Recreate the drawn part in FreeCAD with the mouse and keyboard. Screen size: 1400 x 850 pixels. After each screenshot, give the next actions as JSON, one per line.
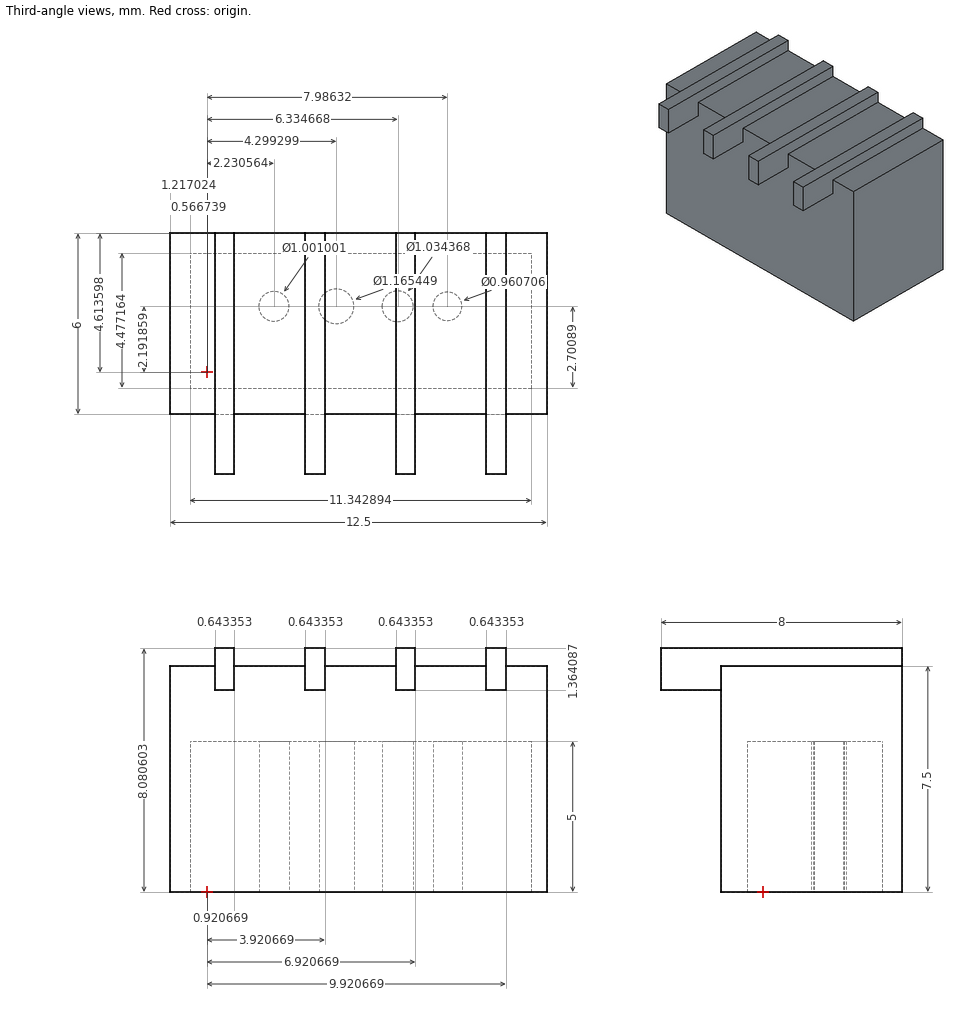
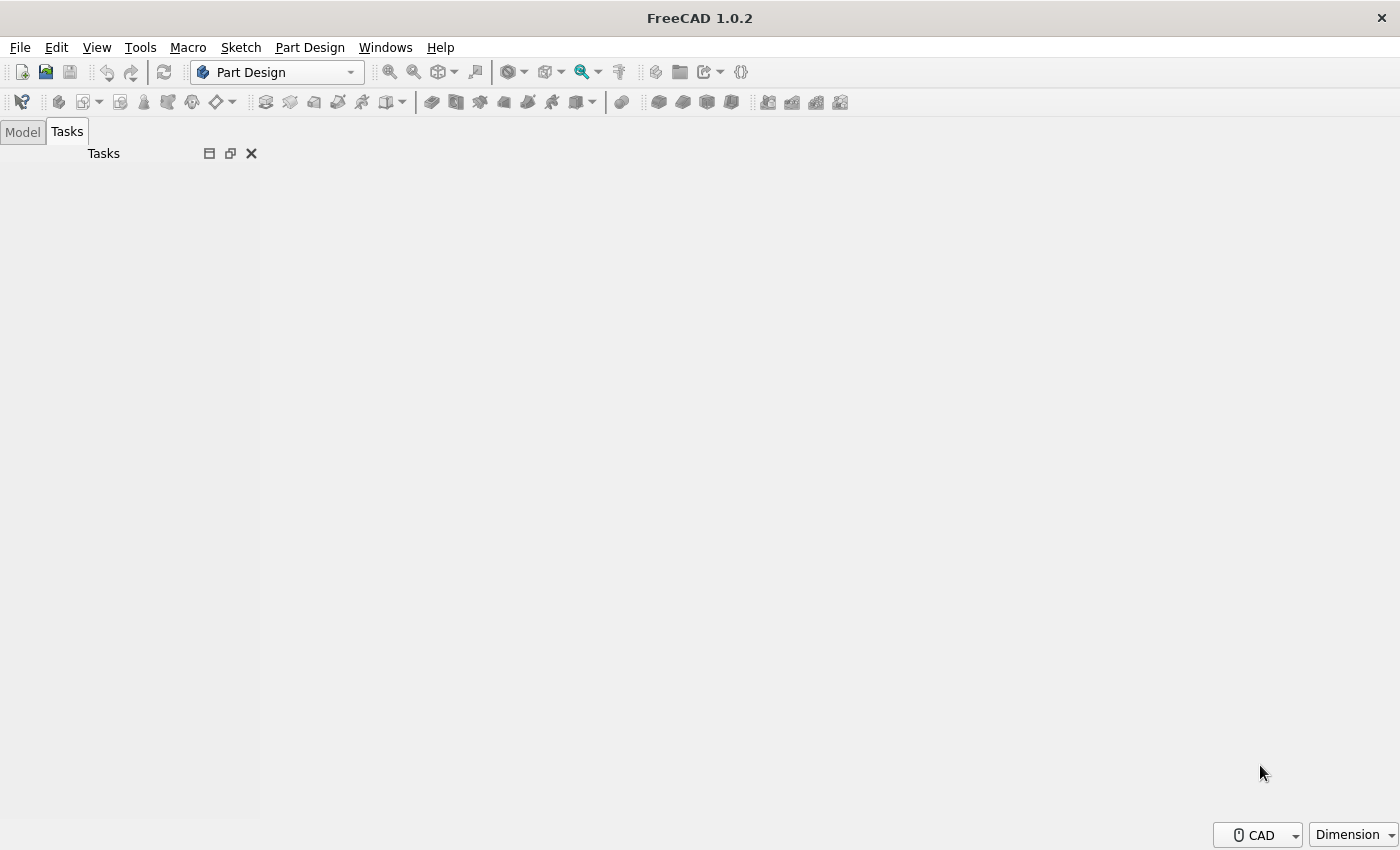
{"action": "key", "text": "ctrl+n"}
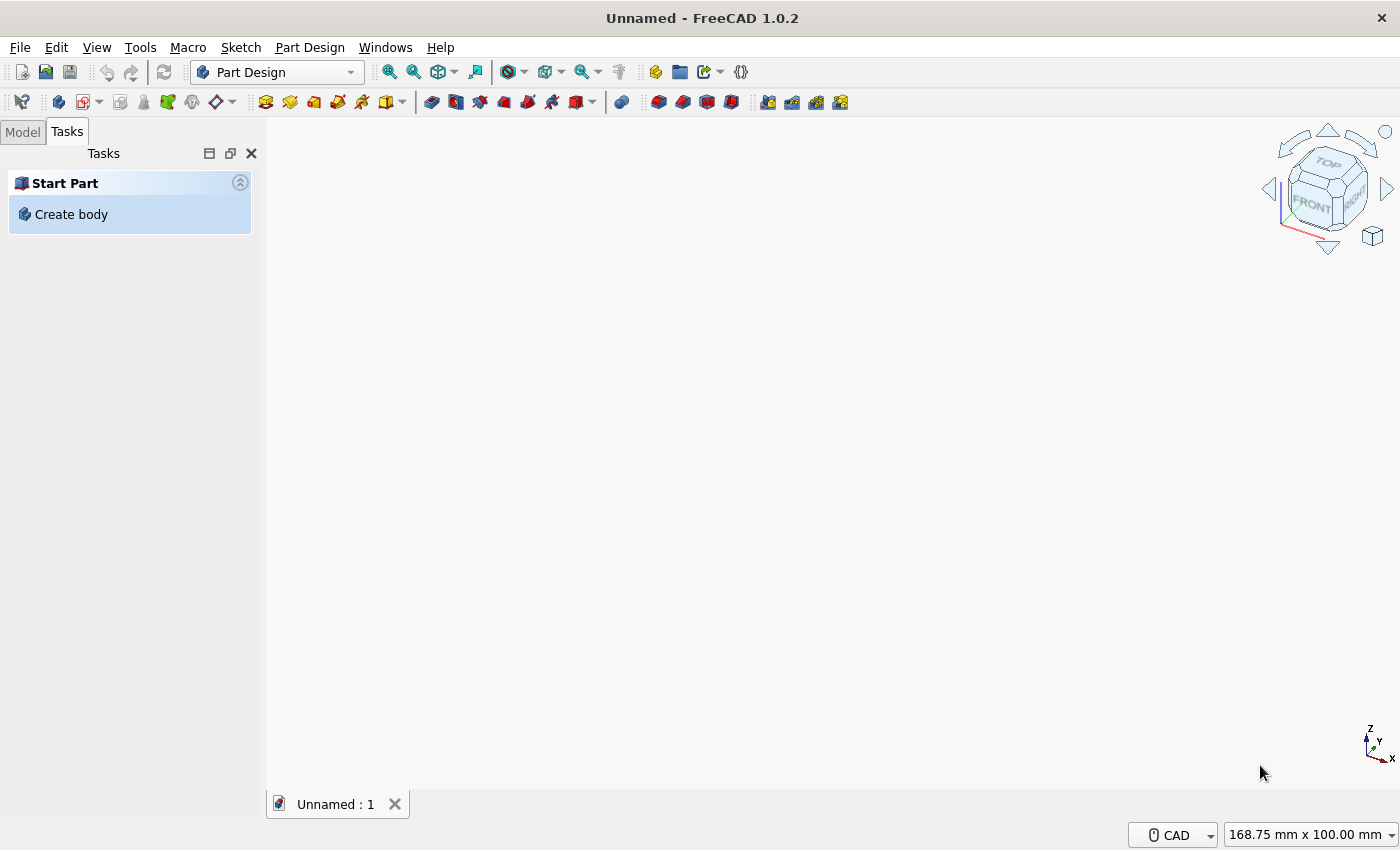
{"action": "left_click", "coordinate": [84, 102]}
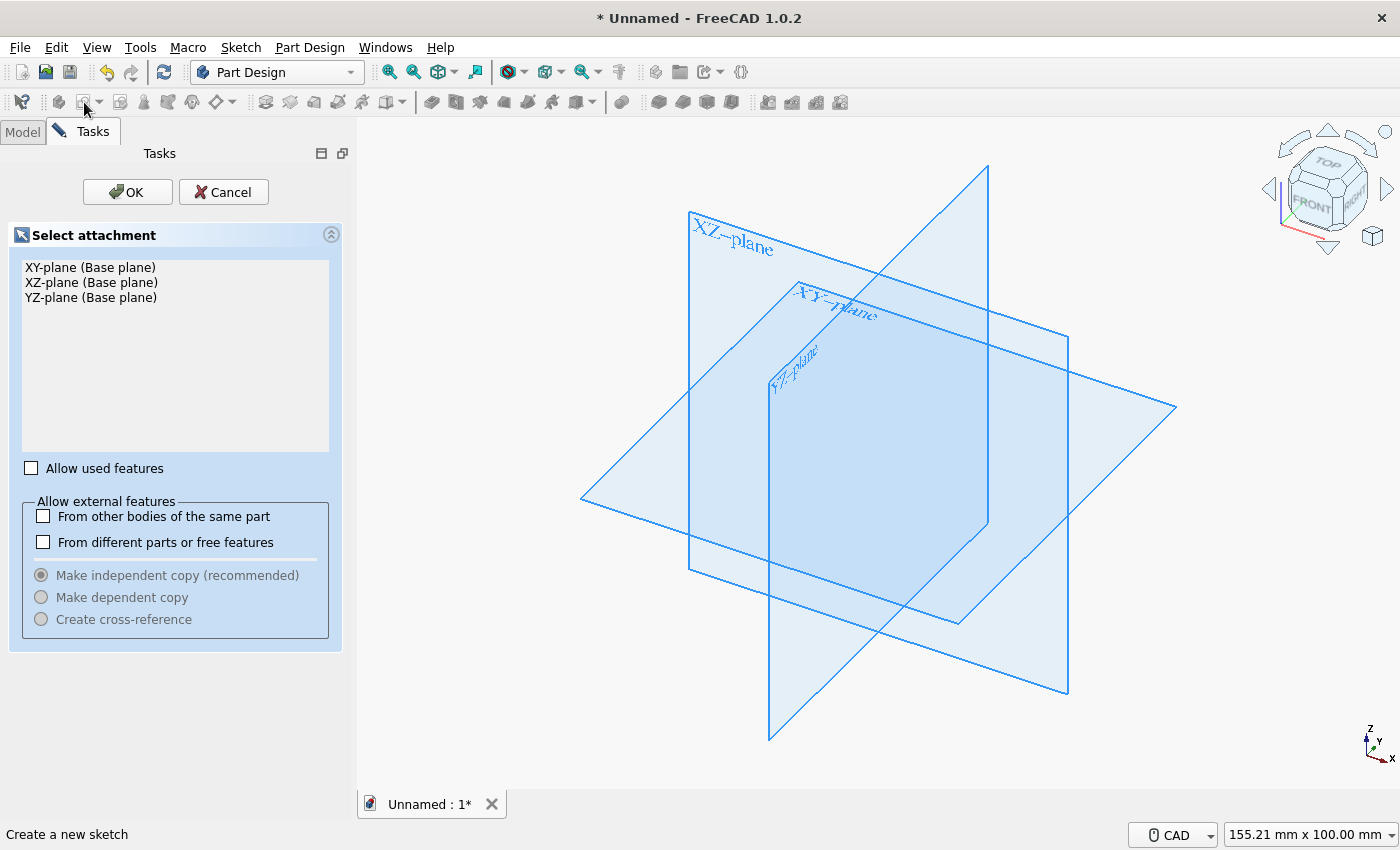
{"action": "left_click", "coordinate": [82, 268]}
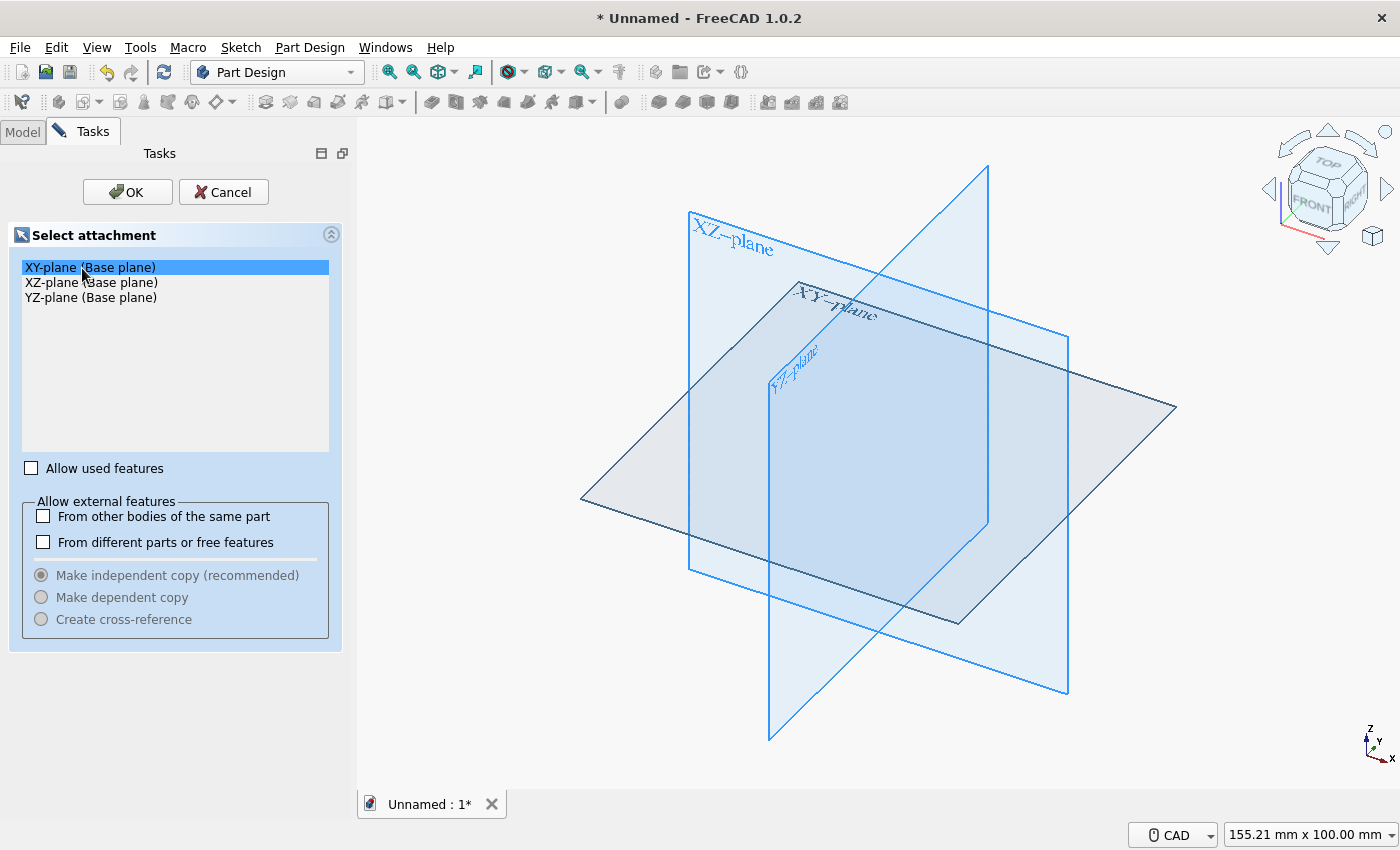
{"action": "left_click", "coordinate": [128, 192]}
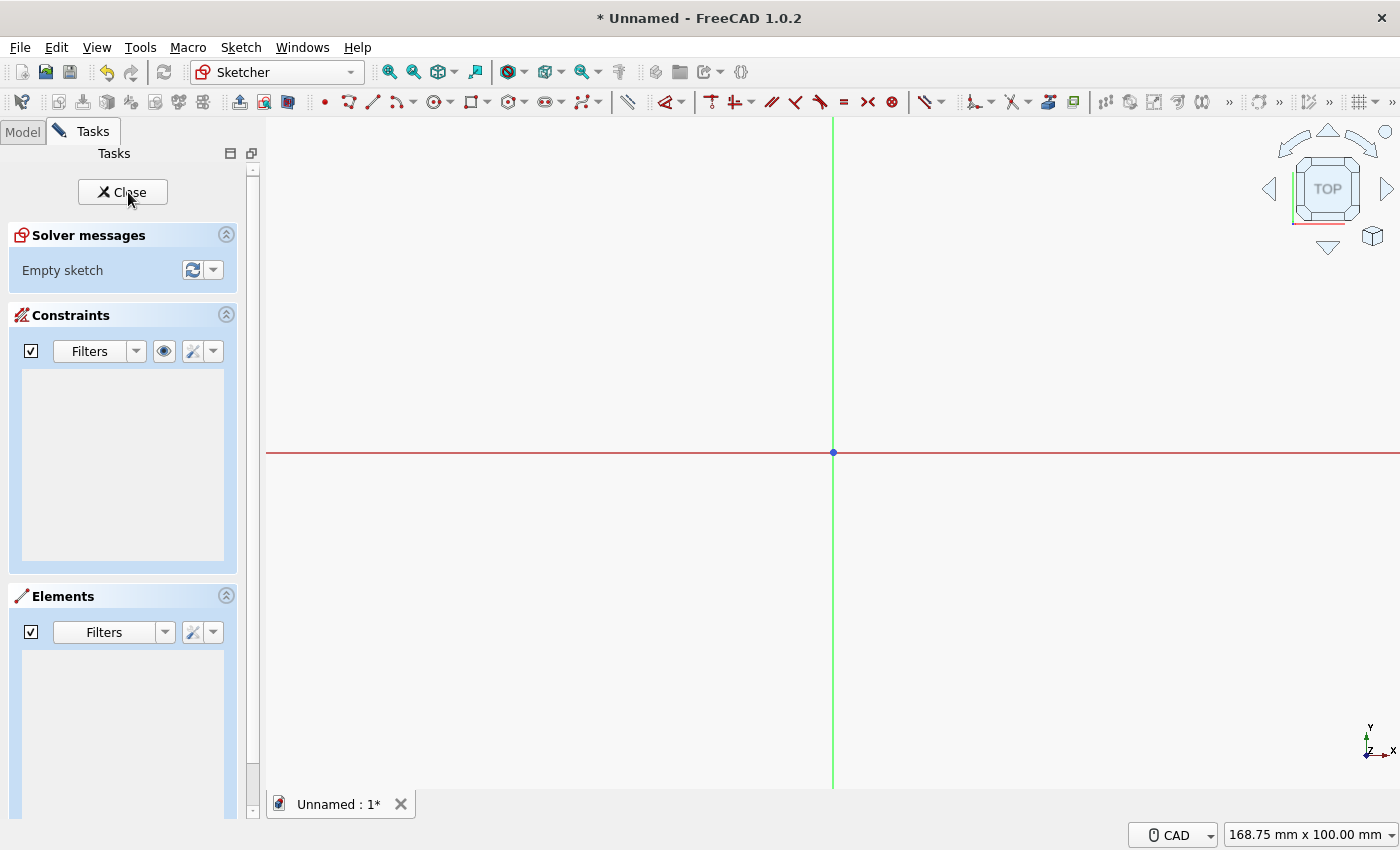
{"action": "scroll", "coordinate": [883, 440], "scroll_direction": "up", "scroll_amount": 10}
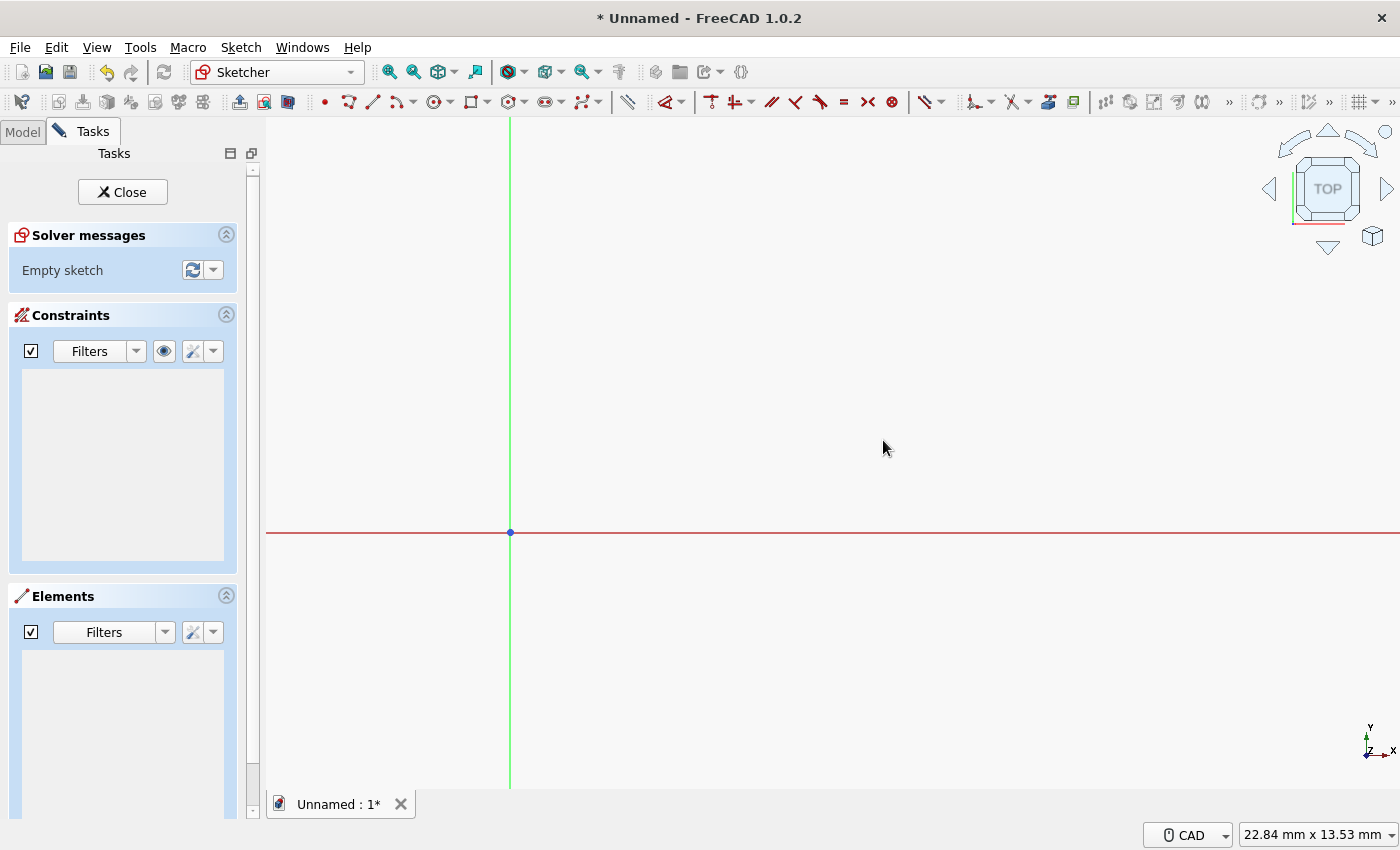
{"action": "key", "text": "g r"}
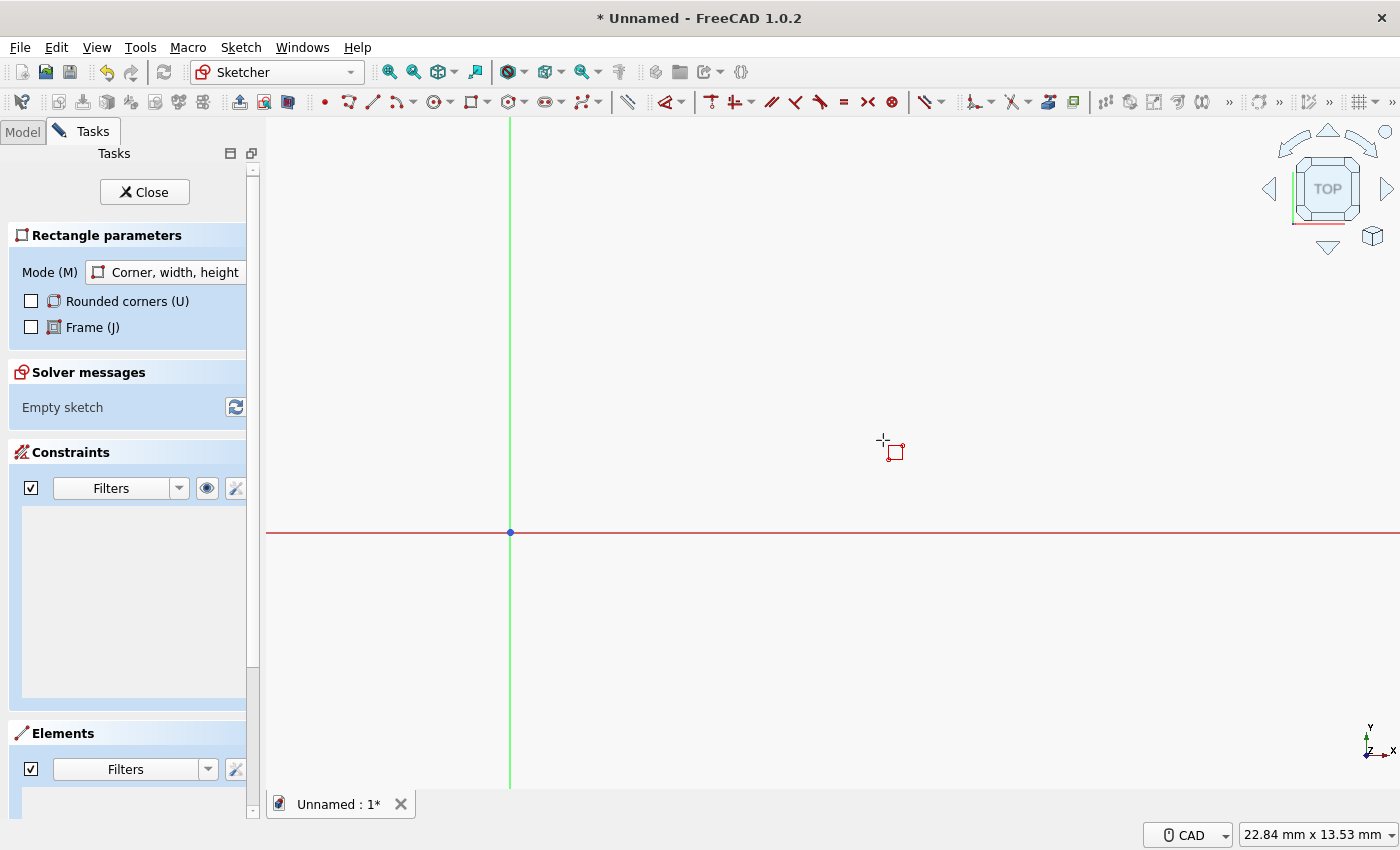
{"action": "left_click", "coordinate": [450, 304]}
{"action": "left_click", "coordinate": [1070, 602]}
{"action": "key", "text": "Escape"}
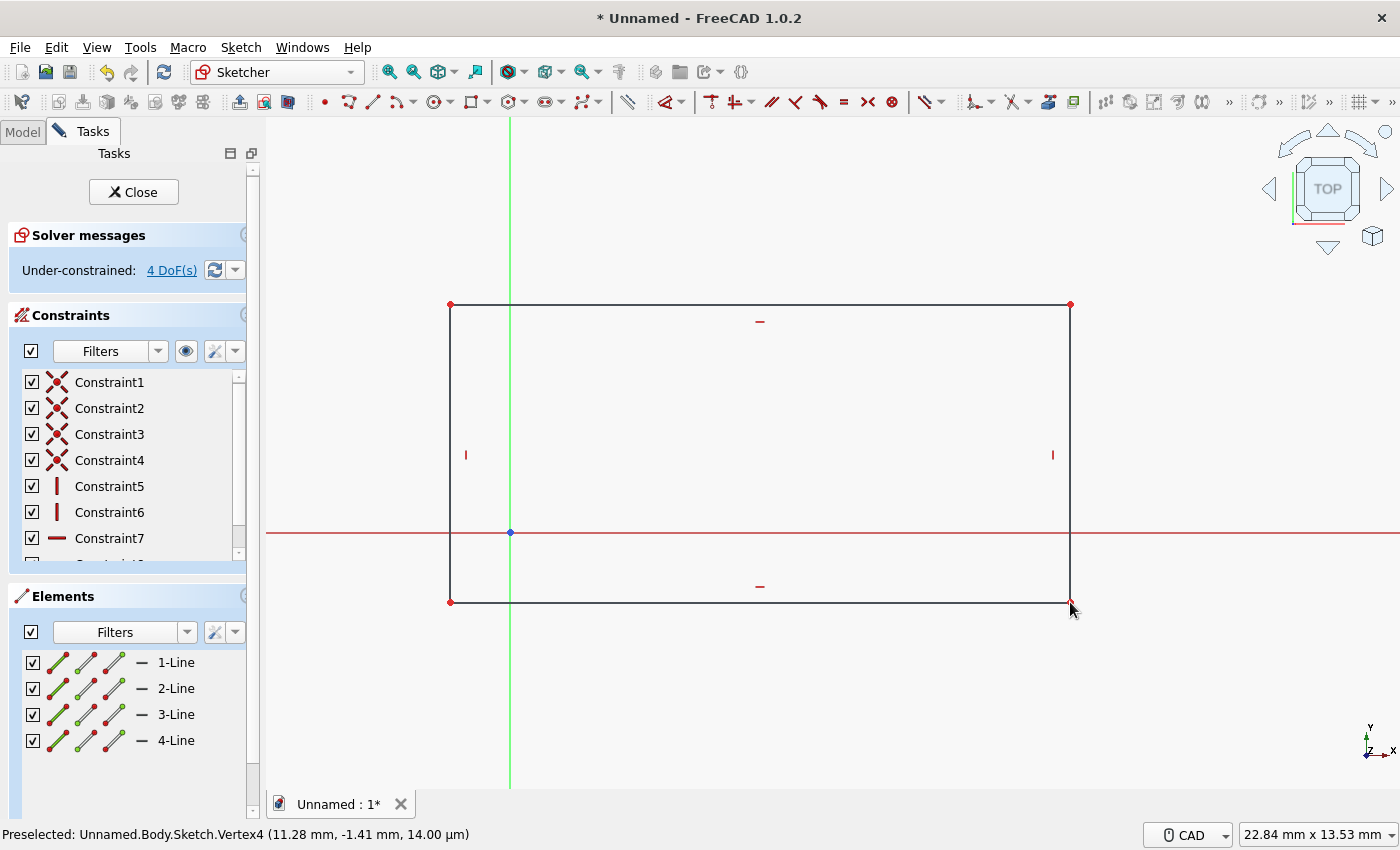
{"action": "left_click", "coordinate": [666, 102]}